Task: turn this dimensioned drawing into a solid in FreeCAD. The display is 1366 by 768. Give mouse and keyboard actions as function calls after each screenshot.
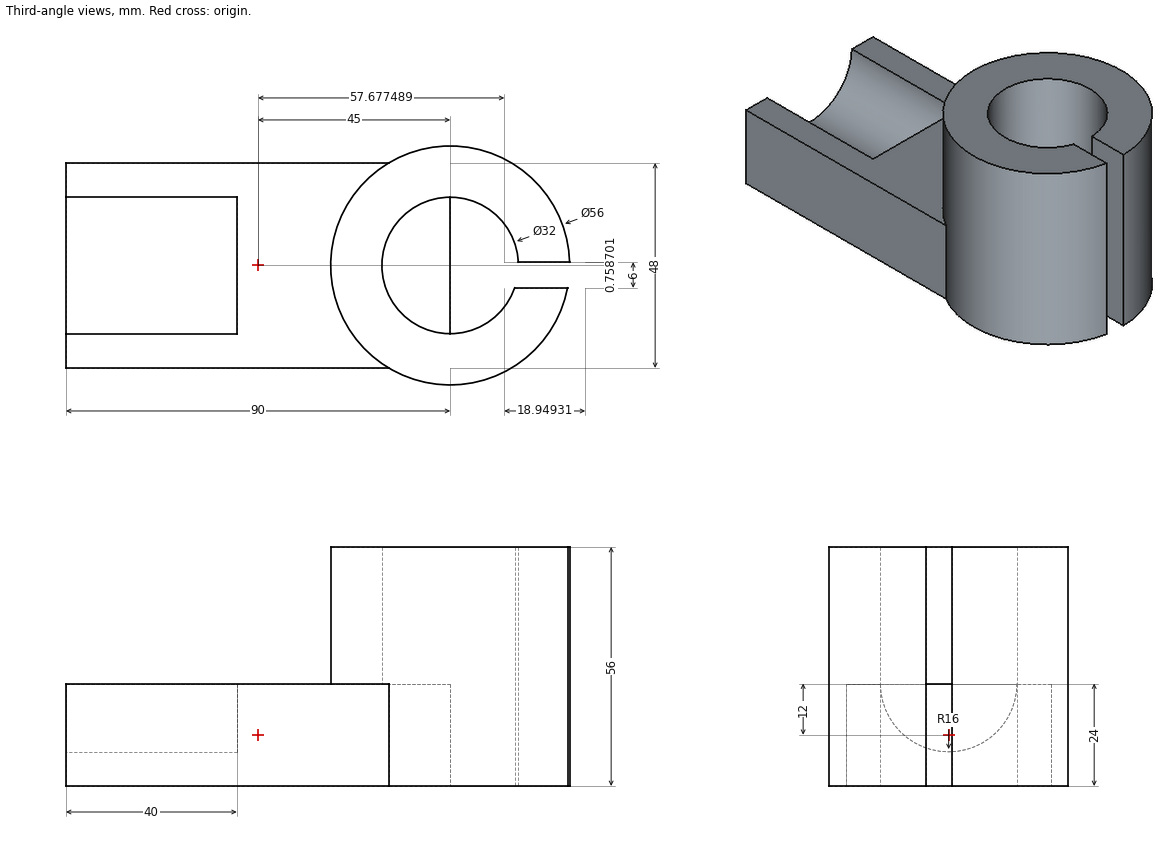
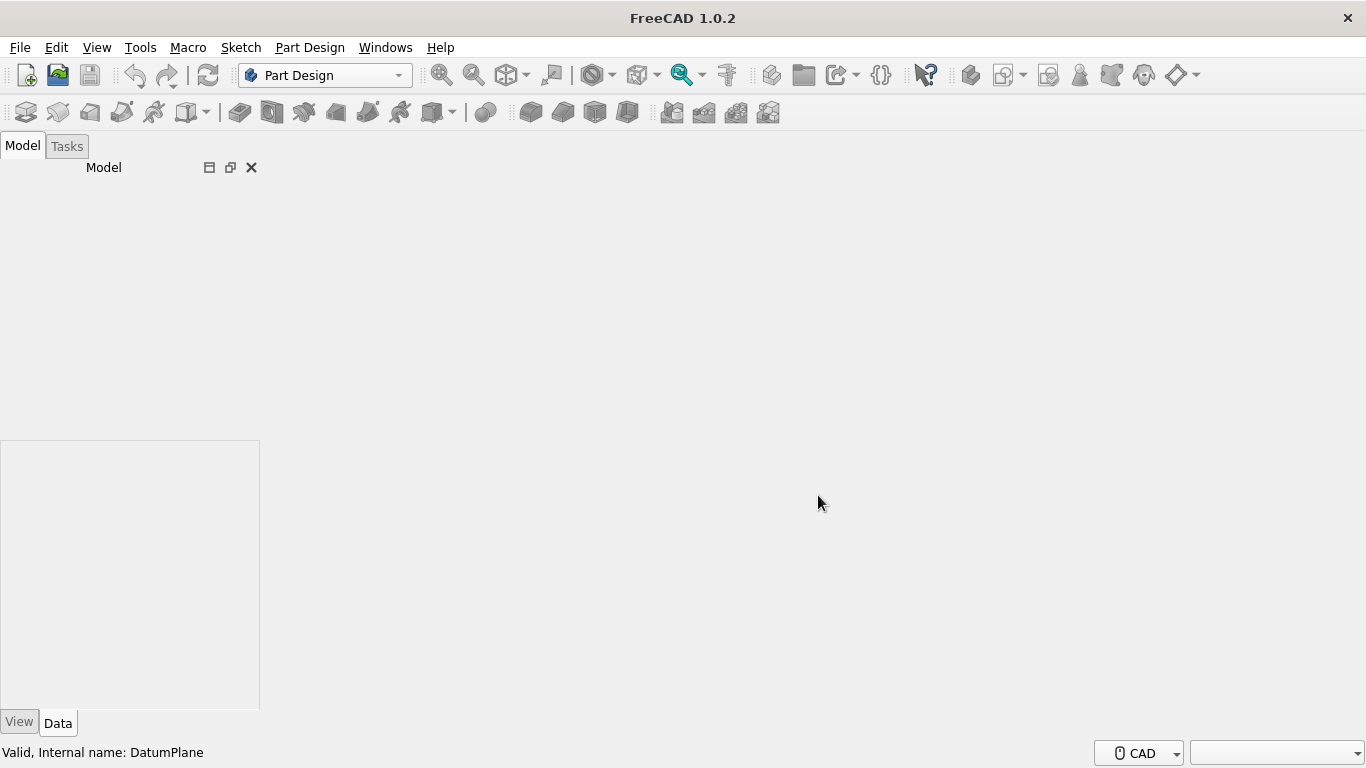
key(ctrl+n)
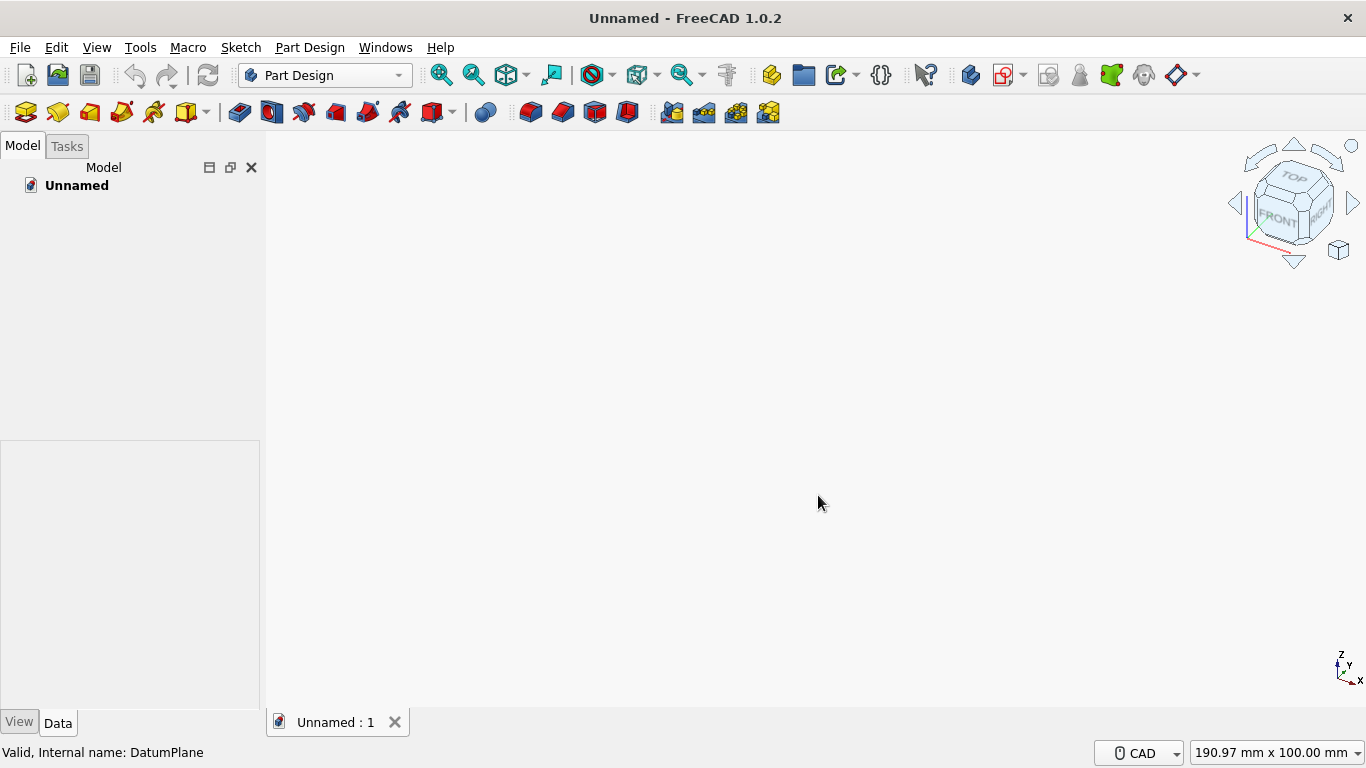
click(1004, 76)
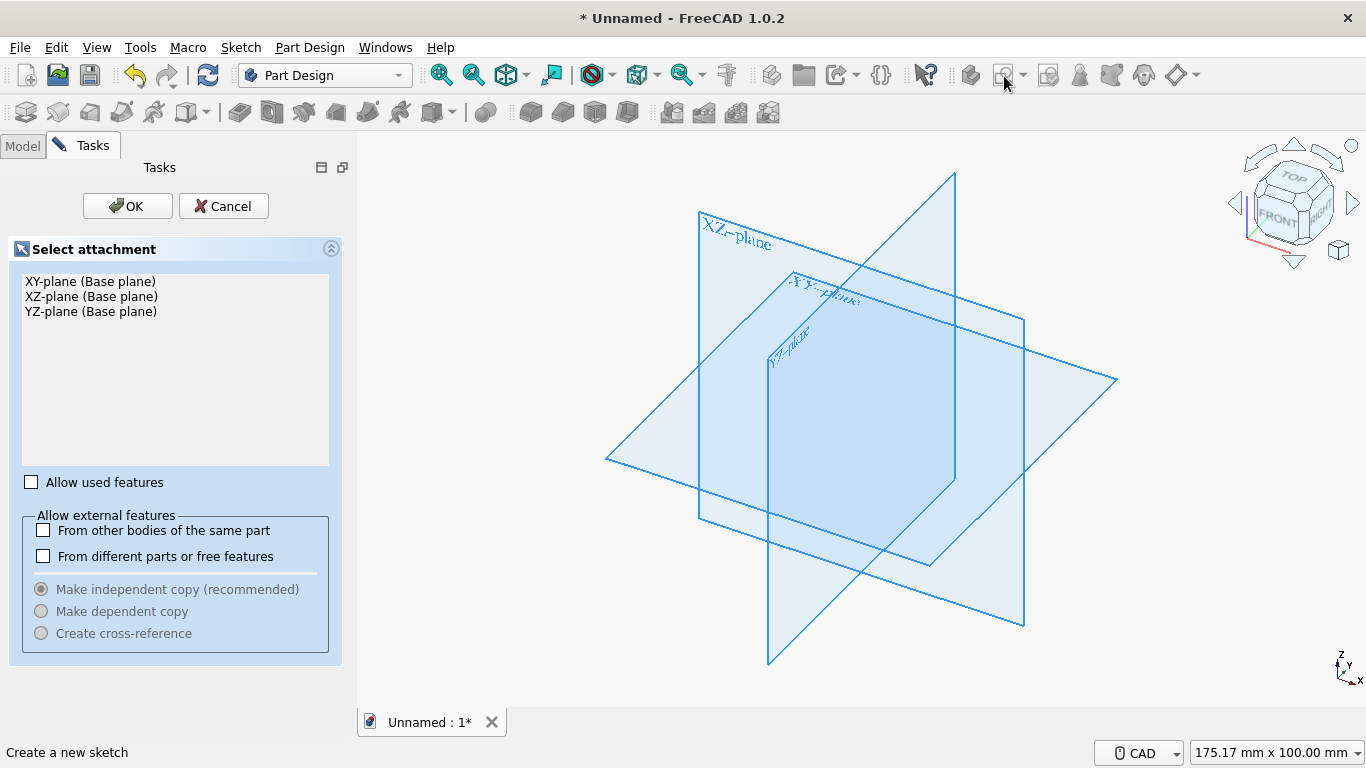
click(82, 282)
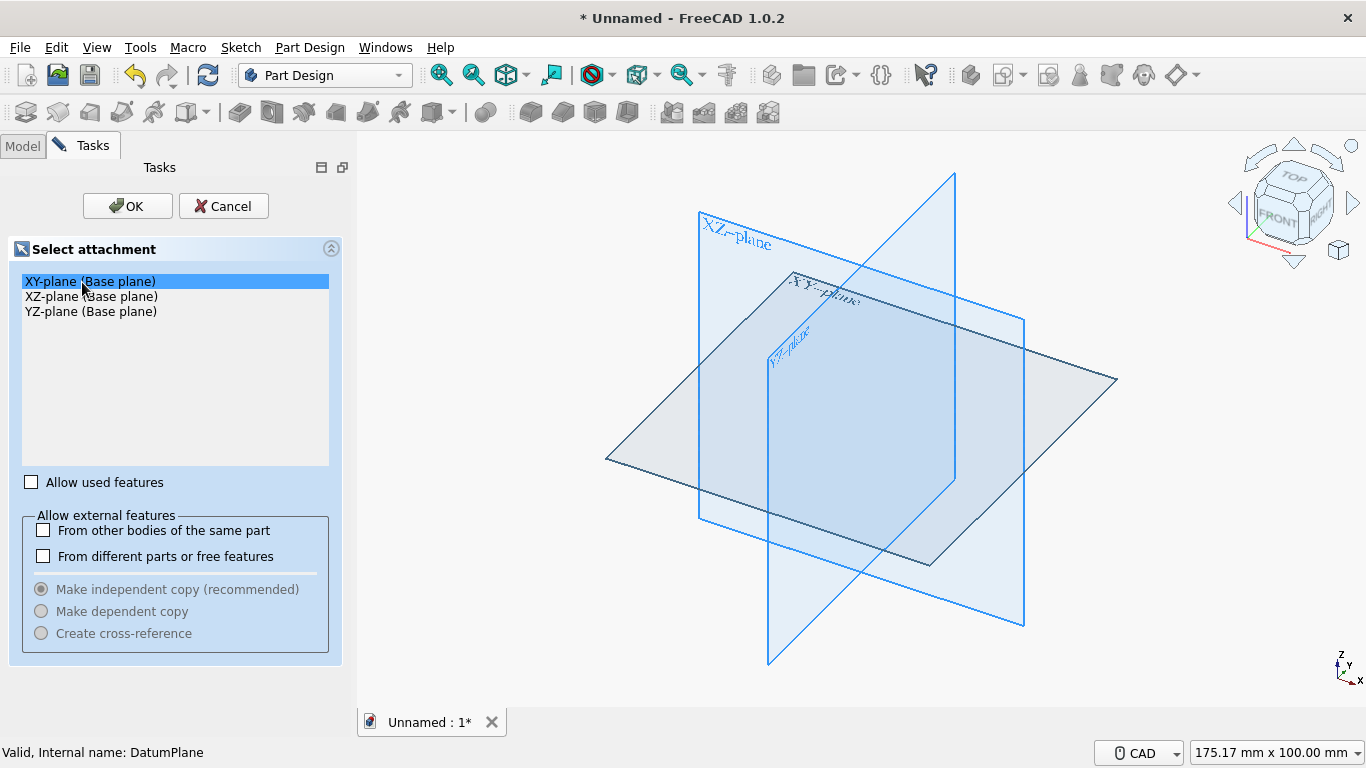
click(128, 206)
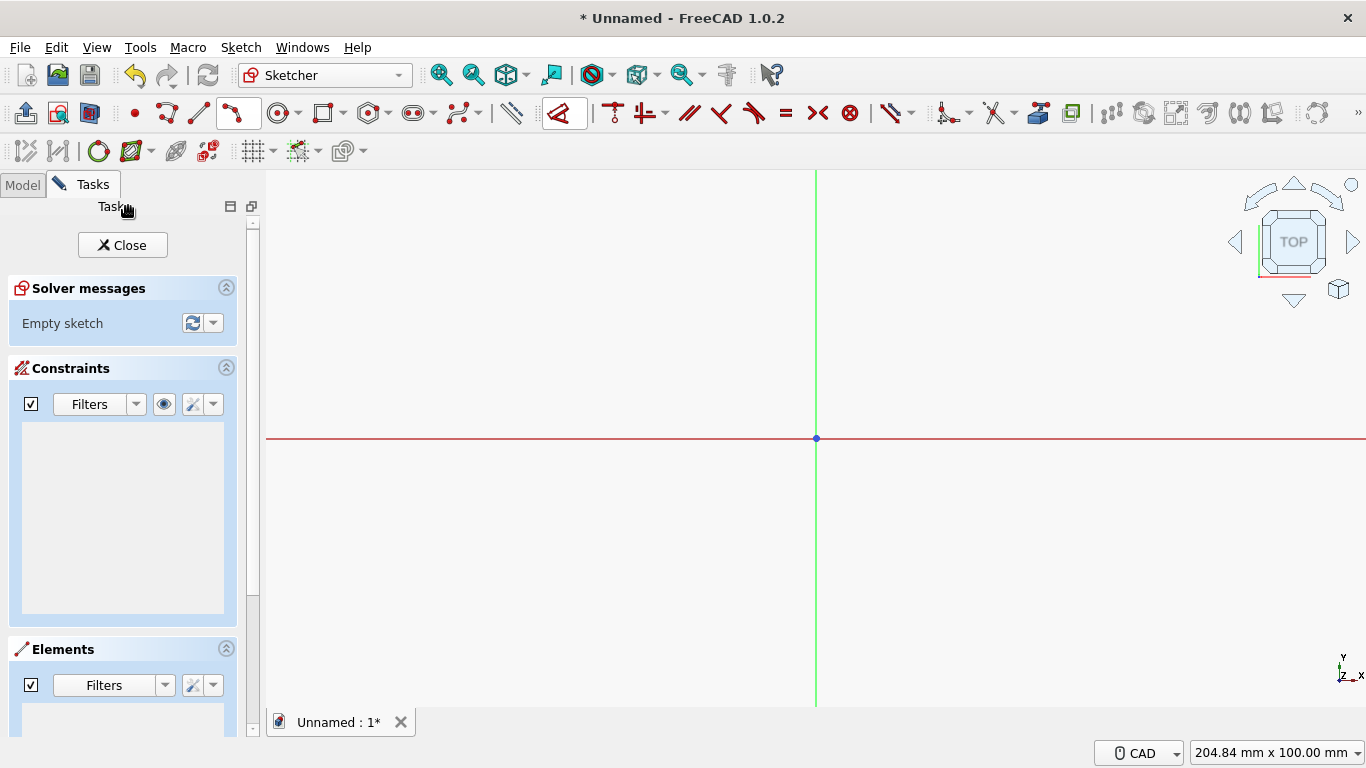
key(g)
key(v)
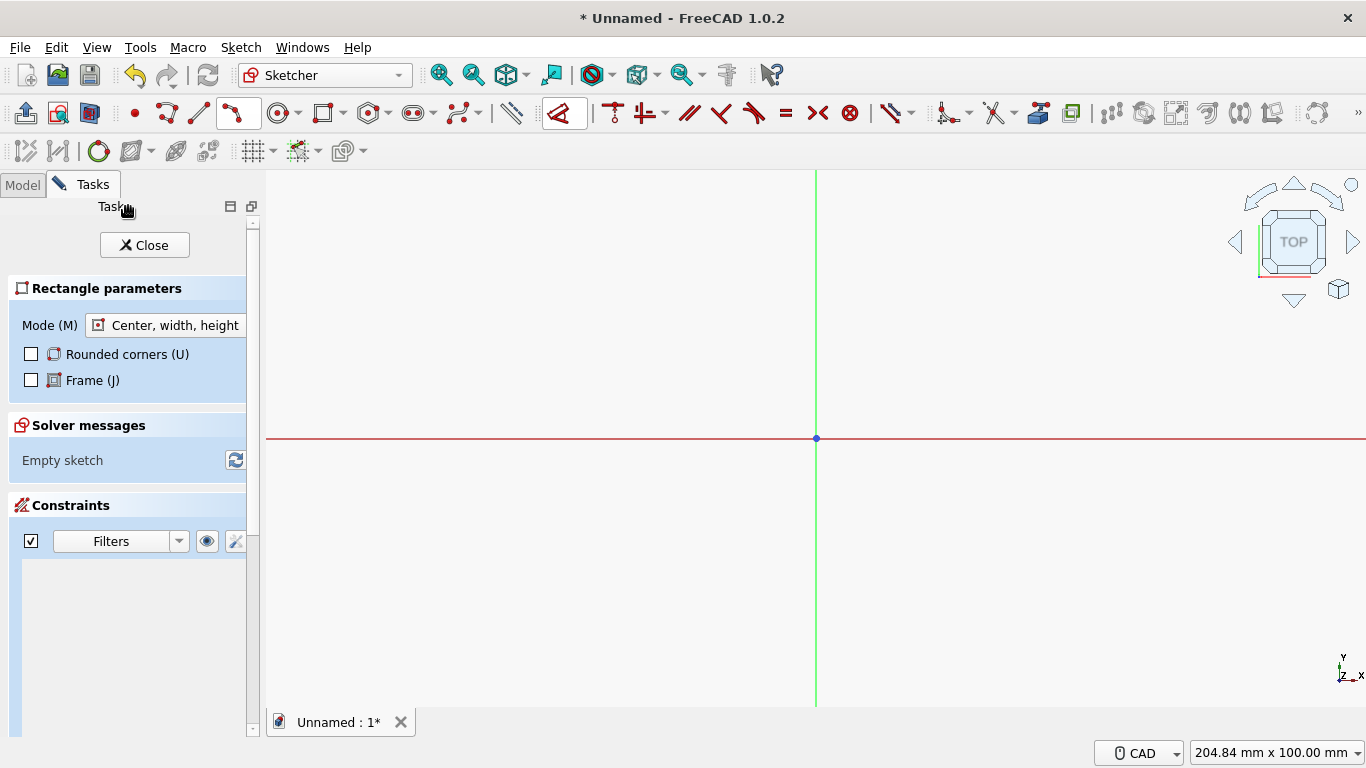
click(816, 438)
move(1058, 310)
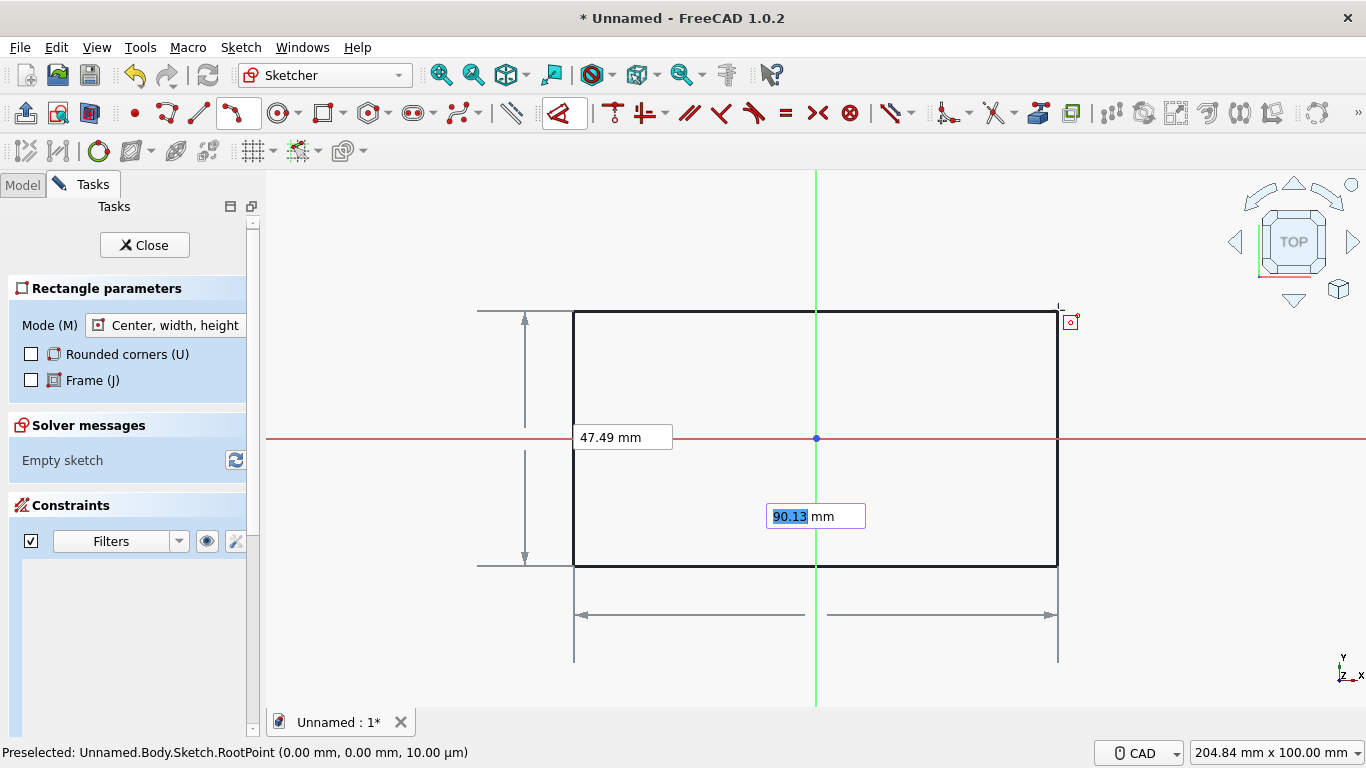
text(90)
key(Tab)
text(48)
key(Return)
key(Escape)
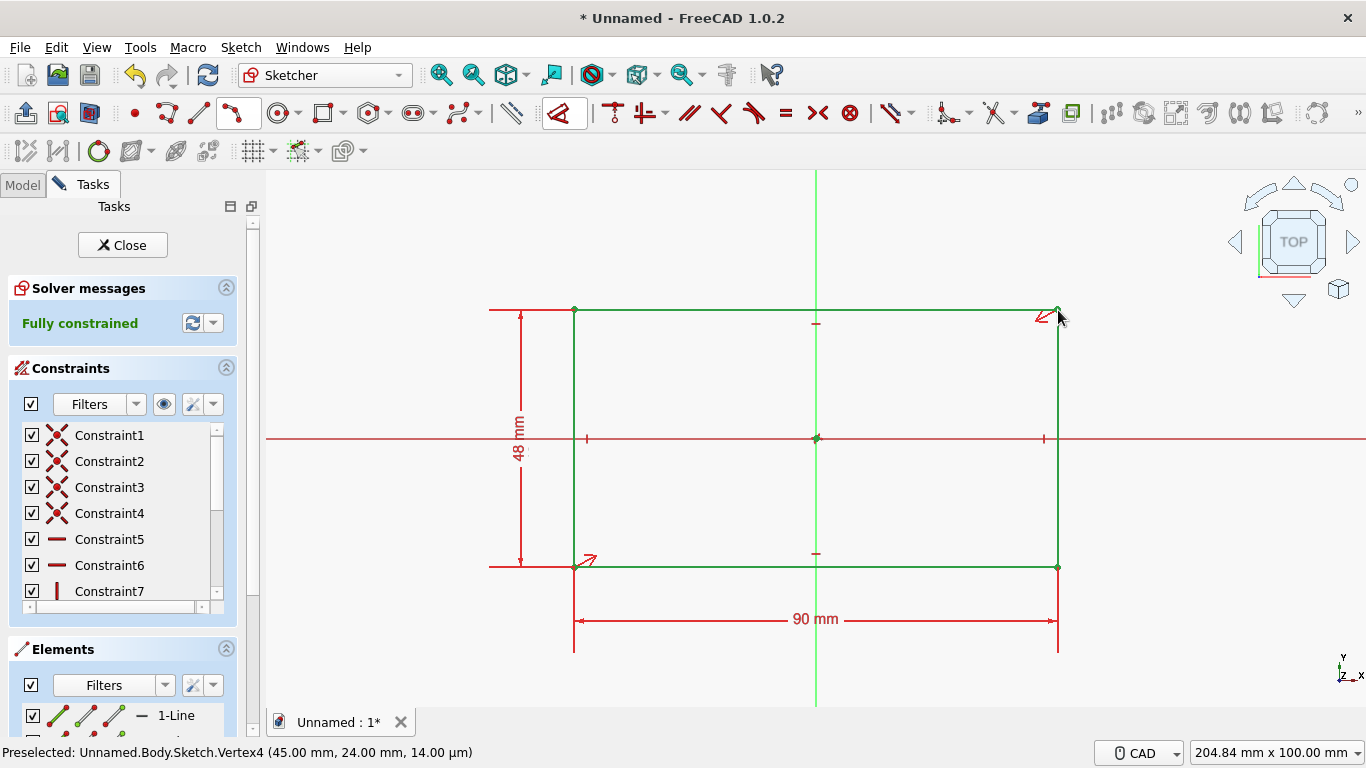
click(123, 245)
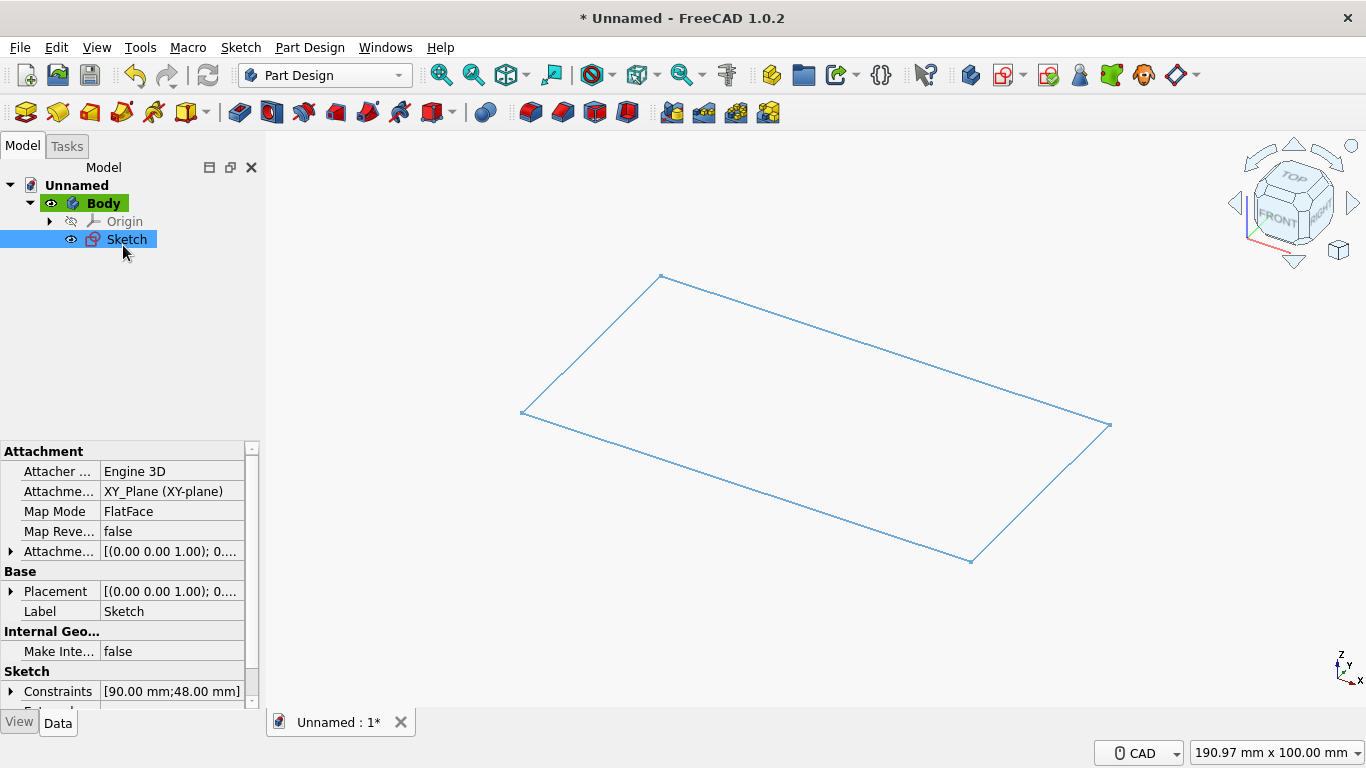
click(26, 112)